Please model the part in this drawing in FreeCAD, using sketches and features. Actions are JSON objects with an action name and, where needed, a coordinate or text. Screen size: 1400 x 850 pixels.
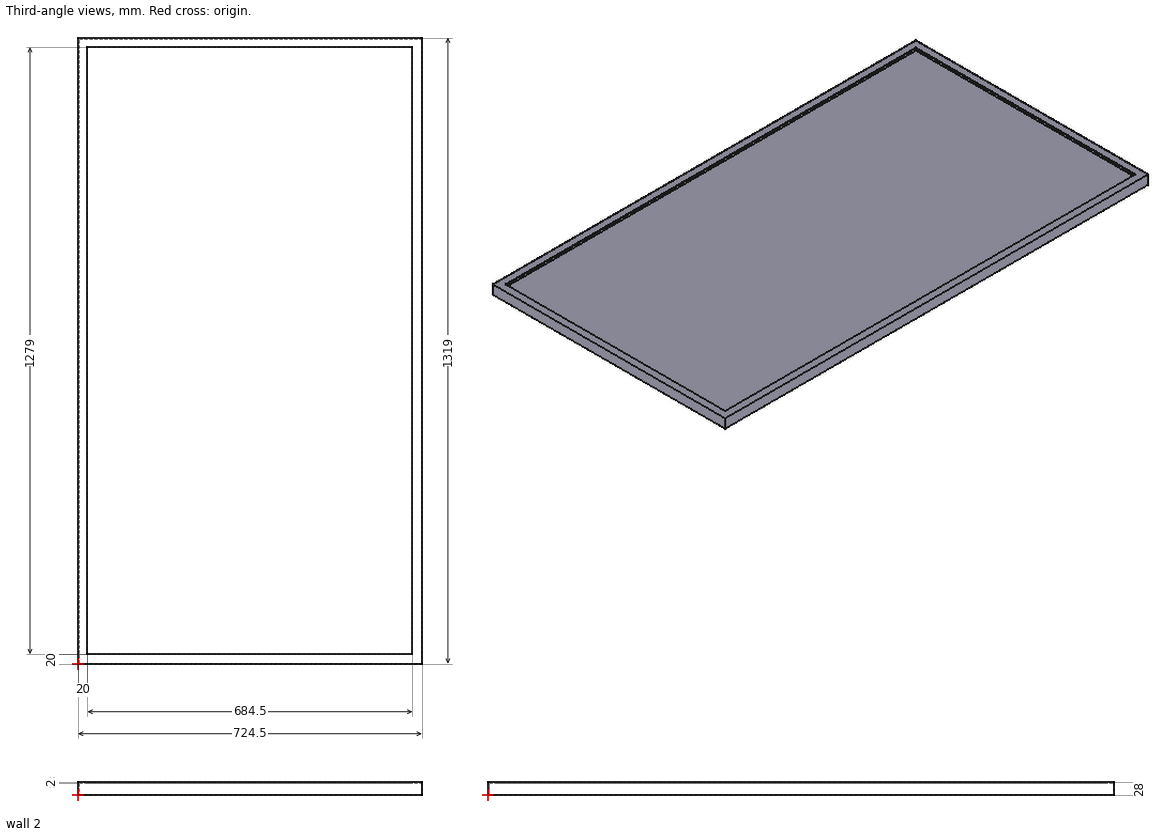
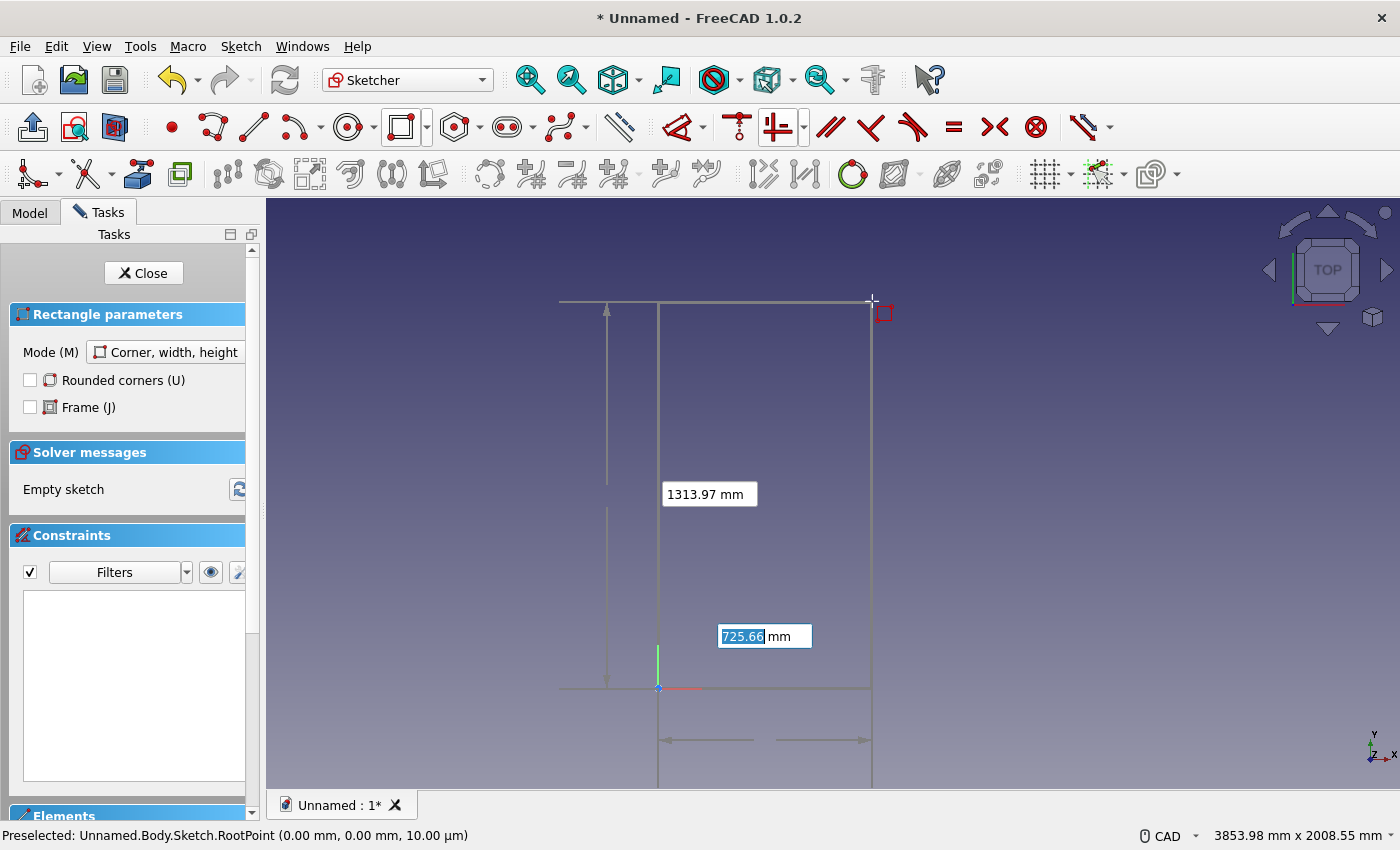
{"action": "type", "text": "724.5"}
{"action": "key", "text": "Tab"}
{"action": "type", "text": "1319"}
{"action": "key", "text": "Return"}
{"action": "key", "text": "Escape"}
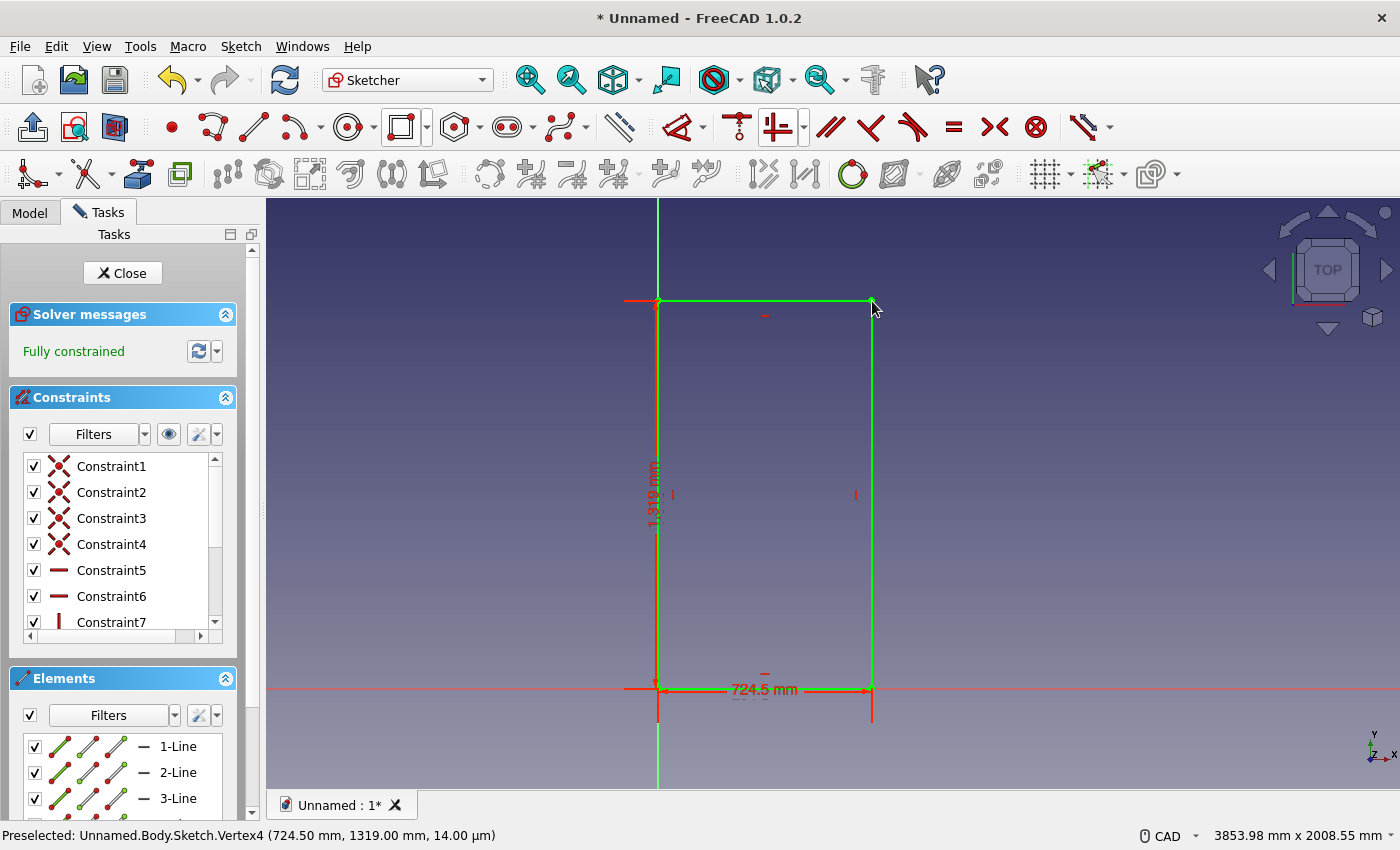
{"action": "left_click", "coordinate": [123, 273]}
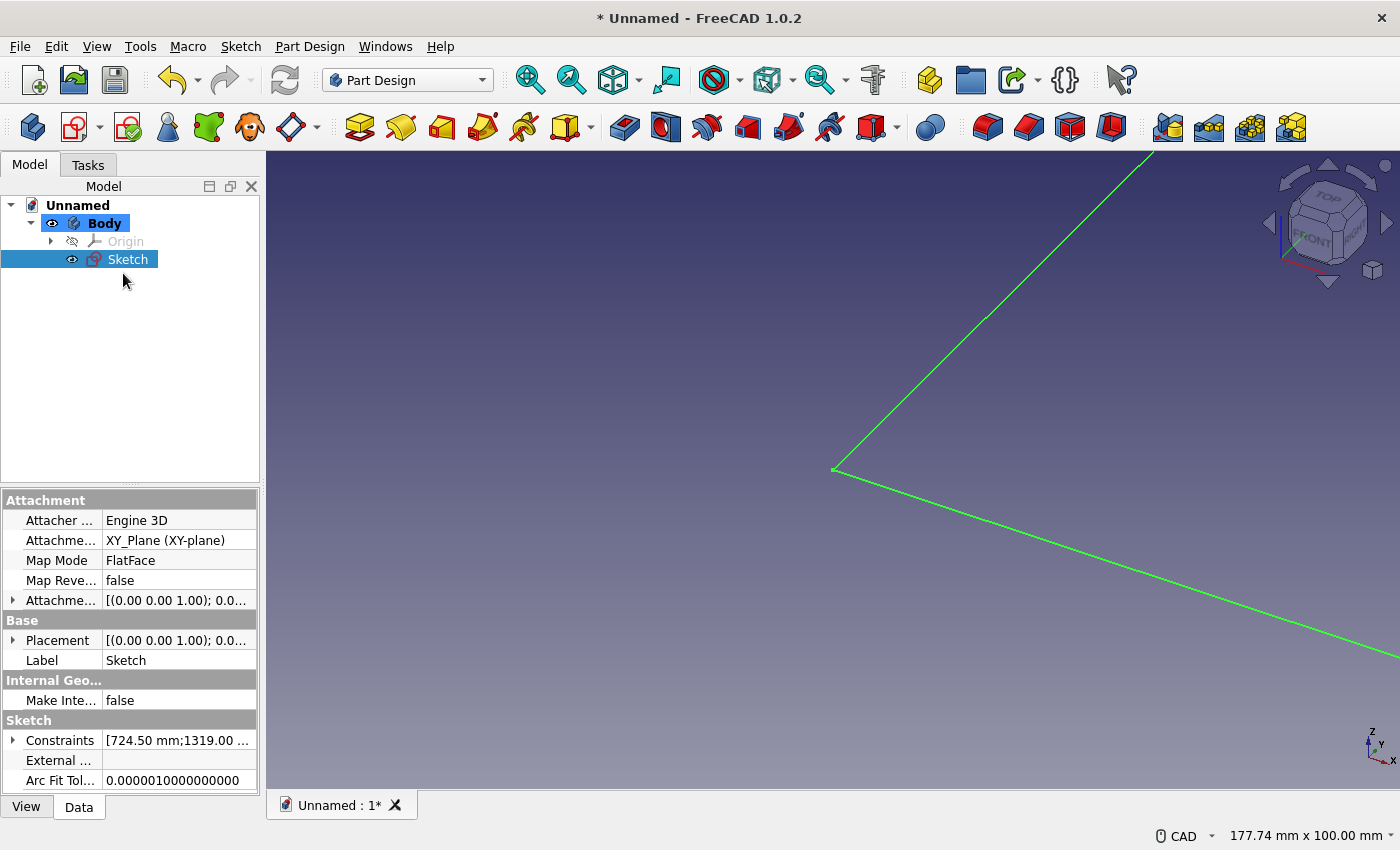
{"action": "left_click", "coordinate": [360, 128]}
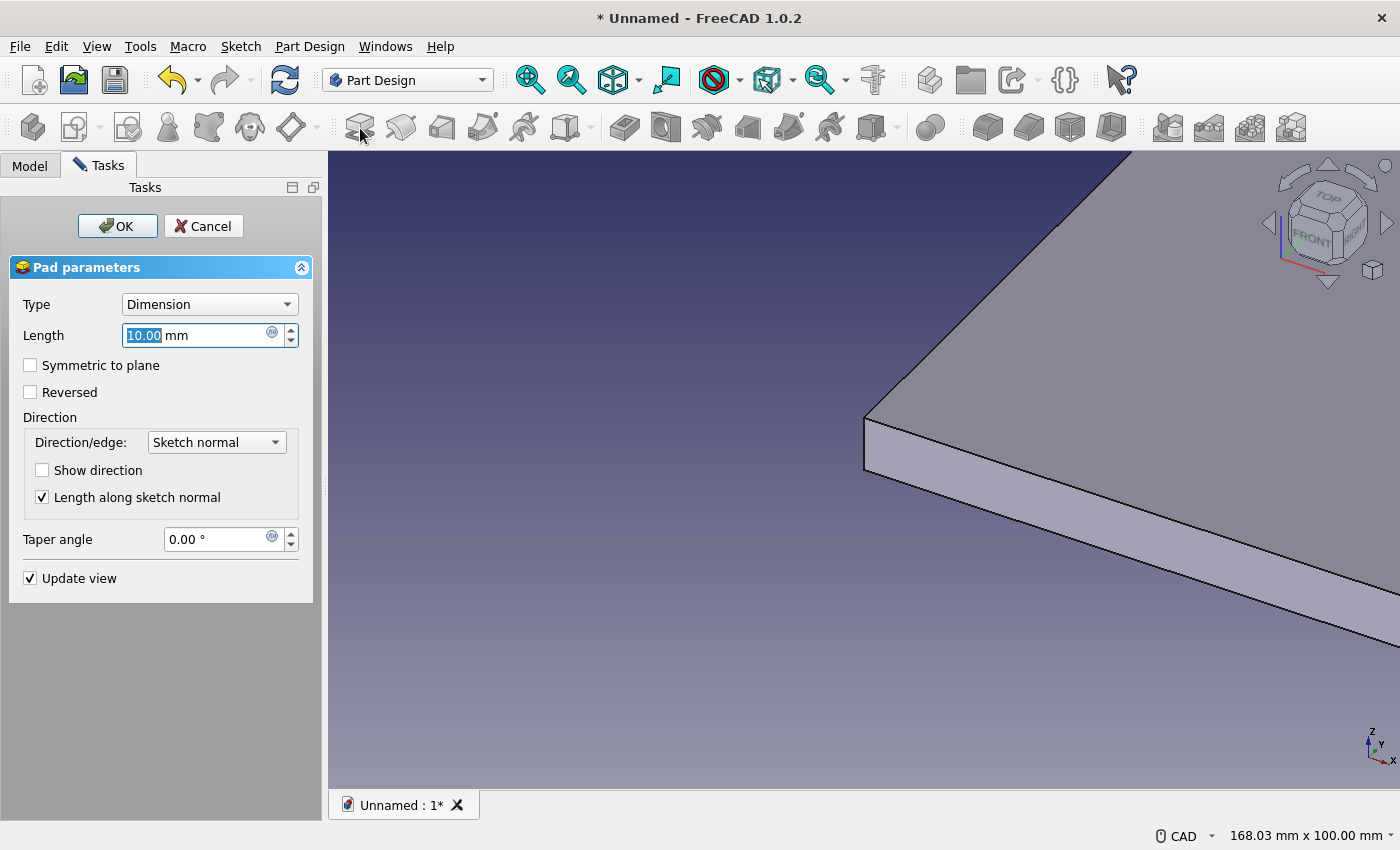
{"action": "type", "text": "28"}
{"action": "key", "text": "Tab"}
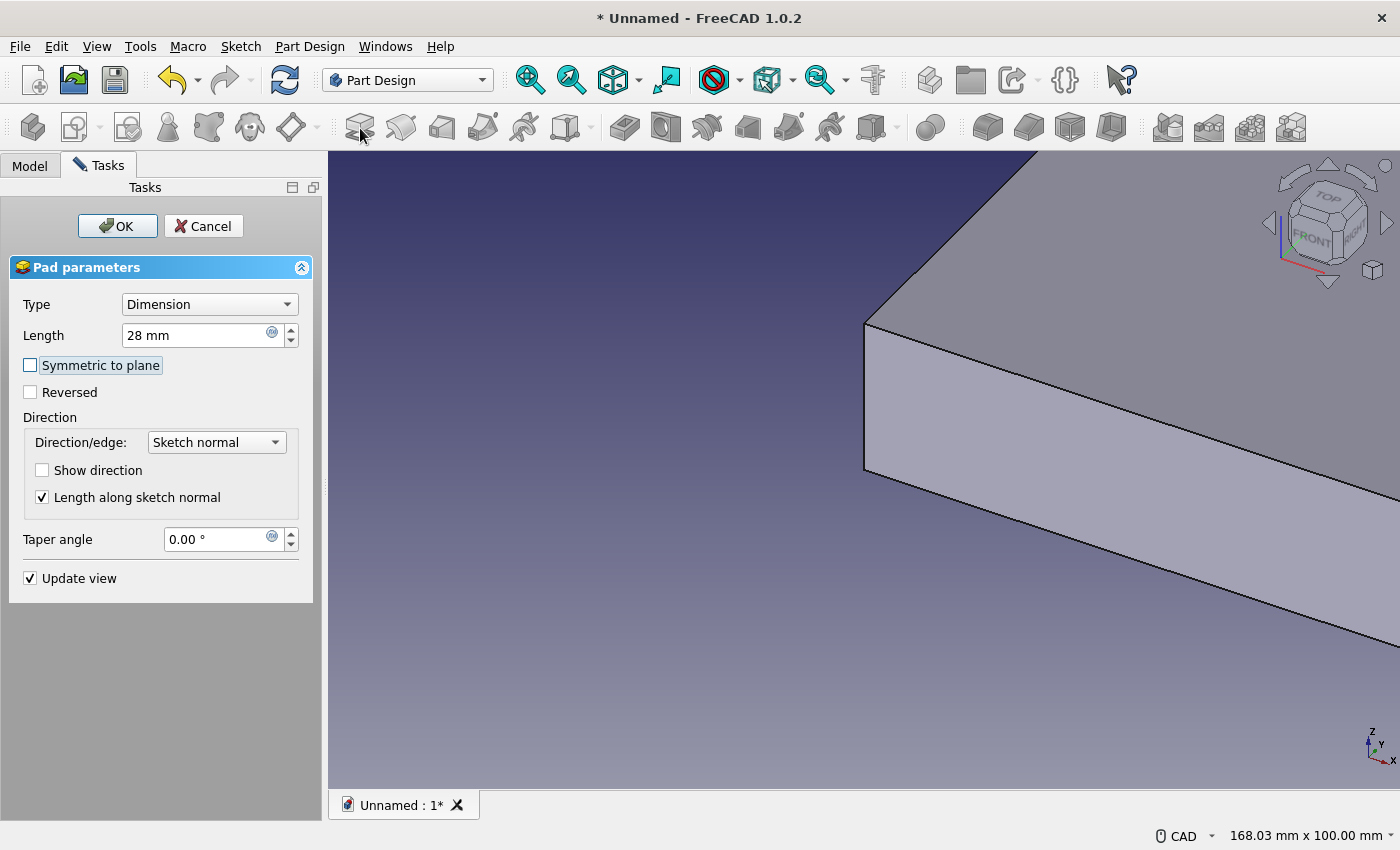
{"action": "left_click", "coordinate": [118, 226]}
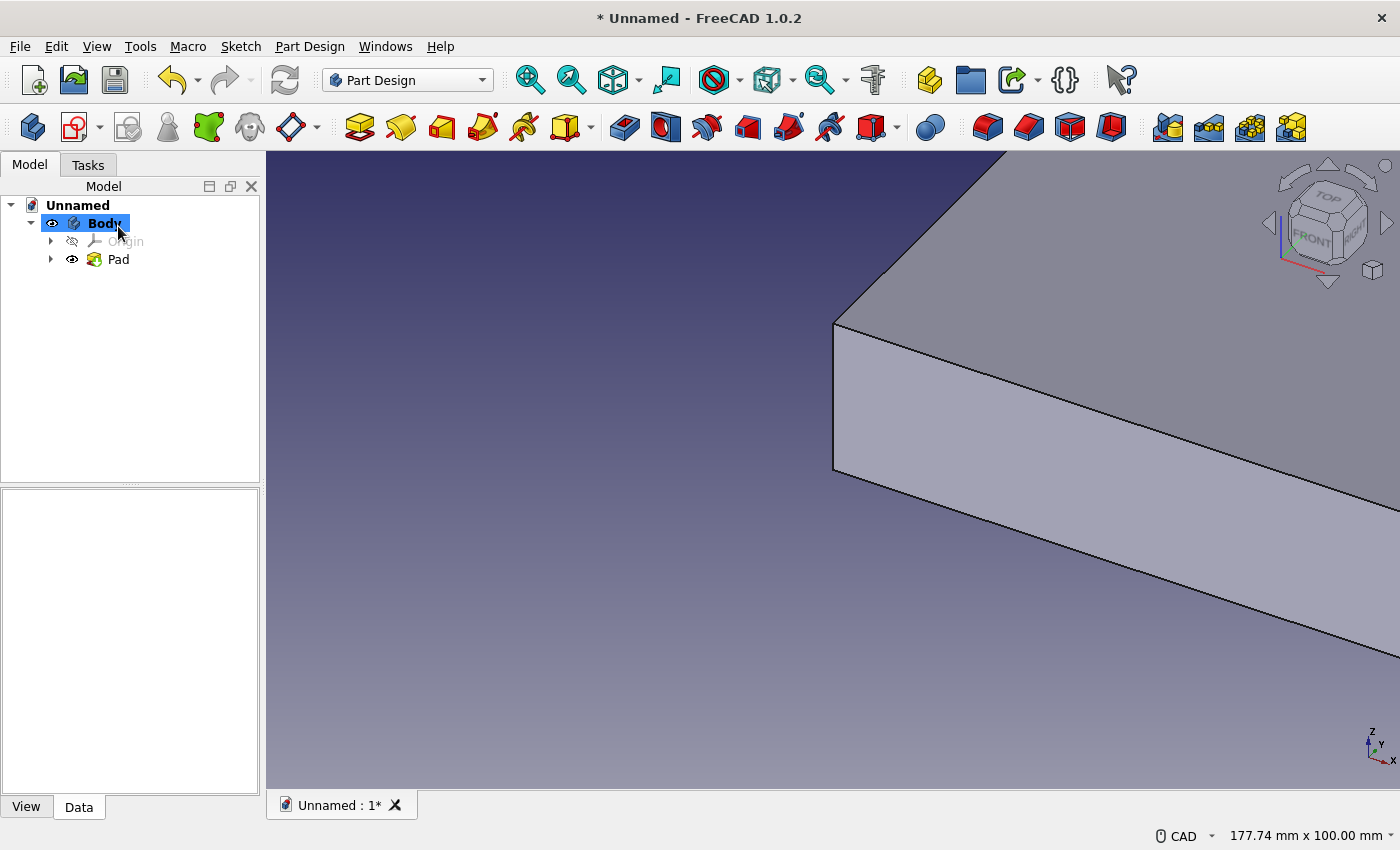
{"action": "left_click", "coordinate": [531, 80]}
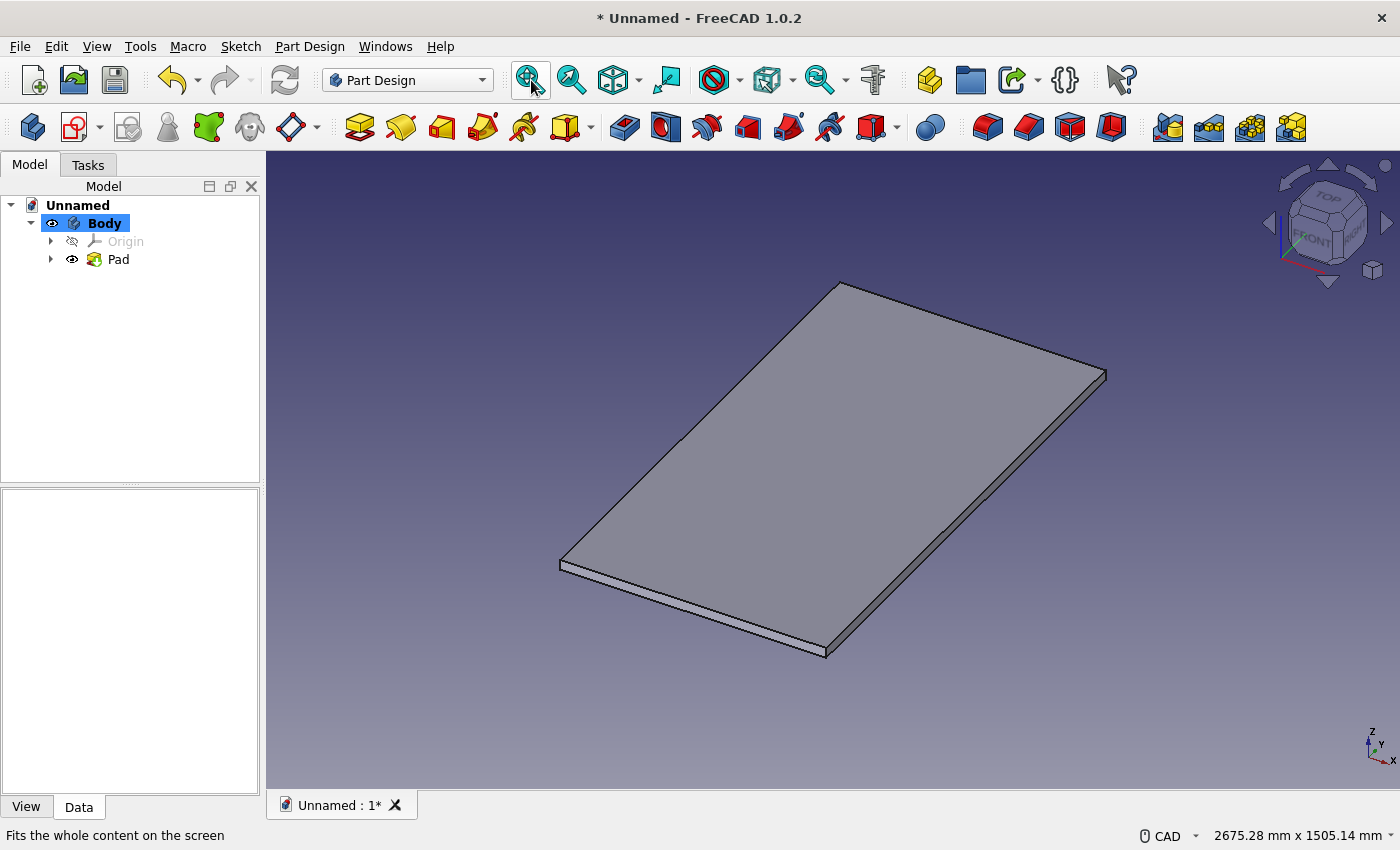
{"action": "left_click", "coordinate": [873, 424]}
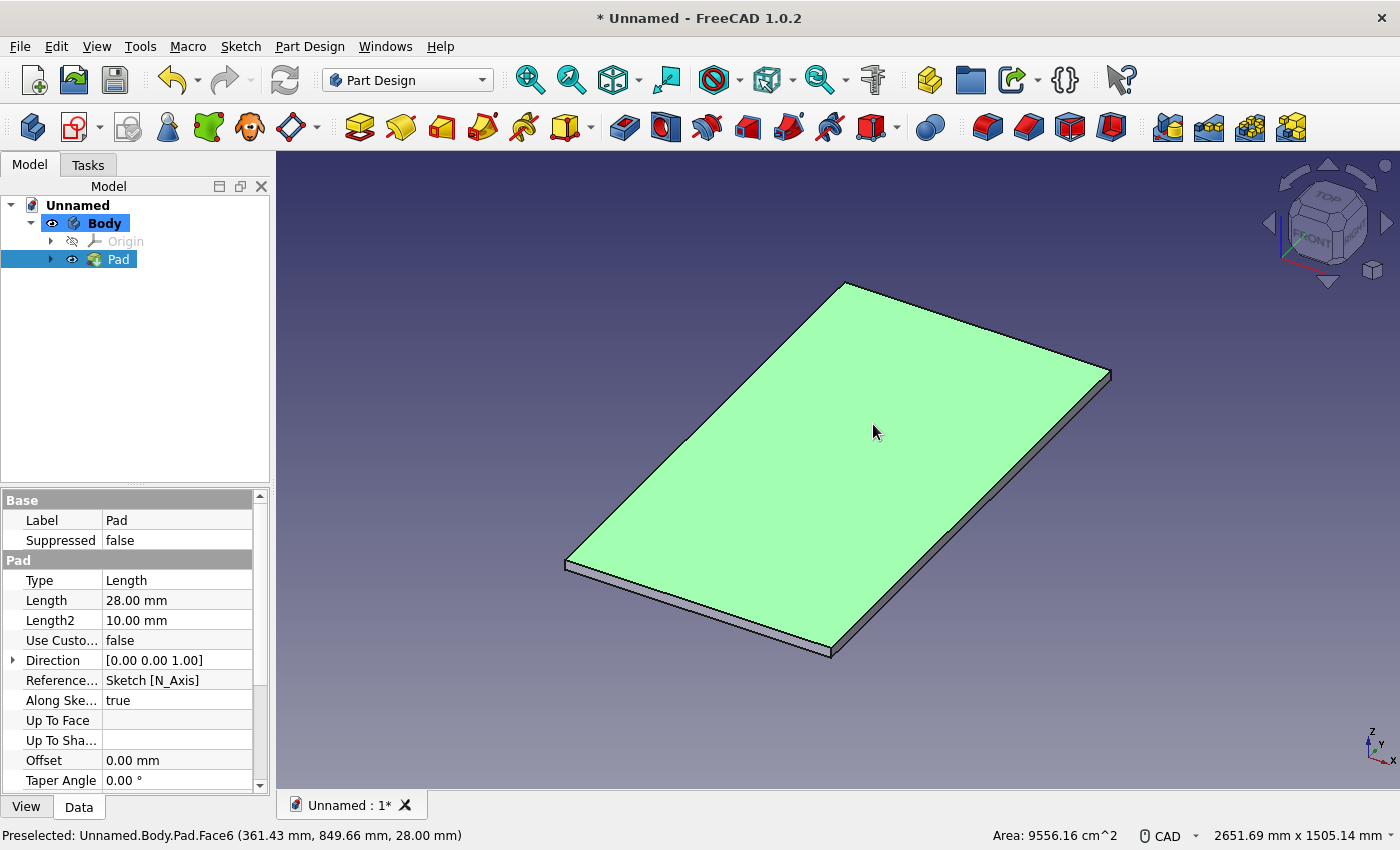
{"action": "left_click", "coordinate": [1111, 128]}